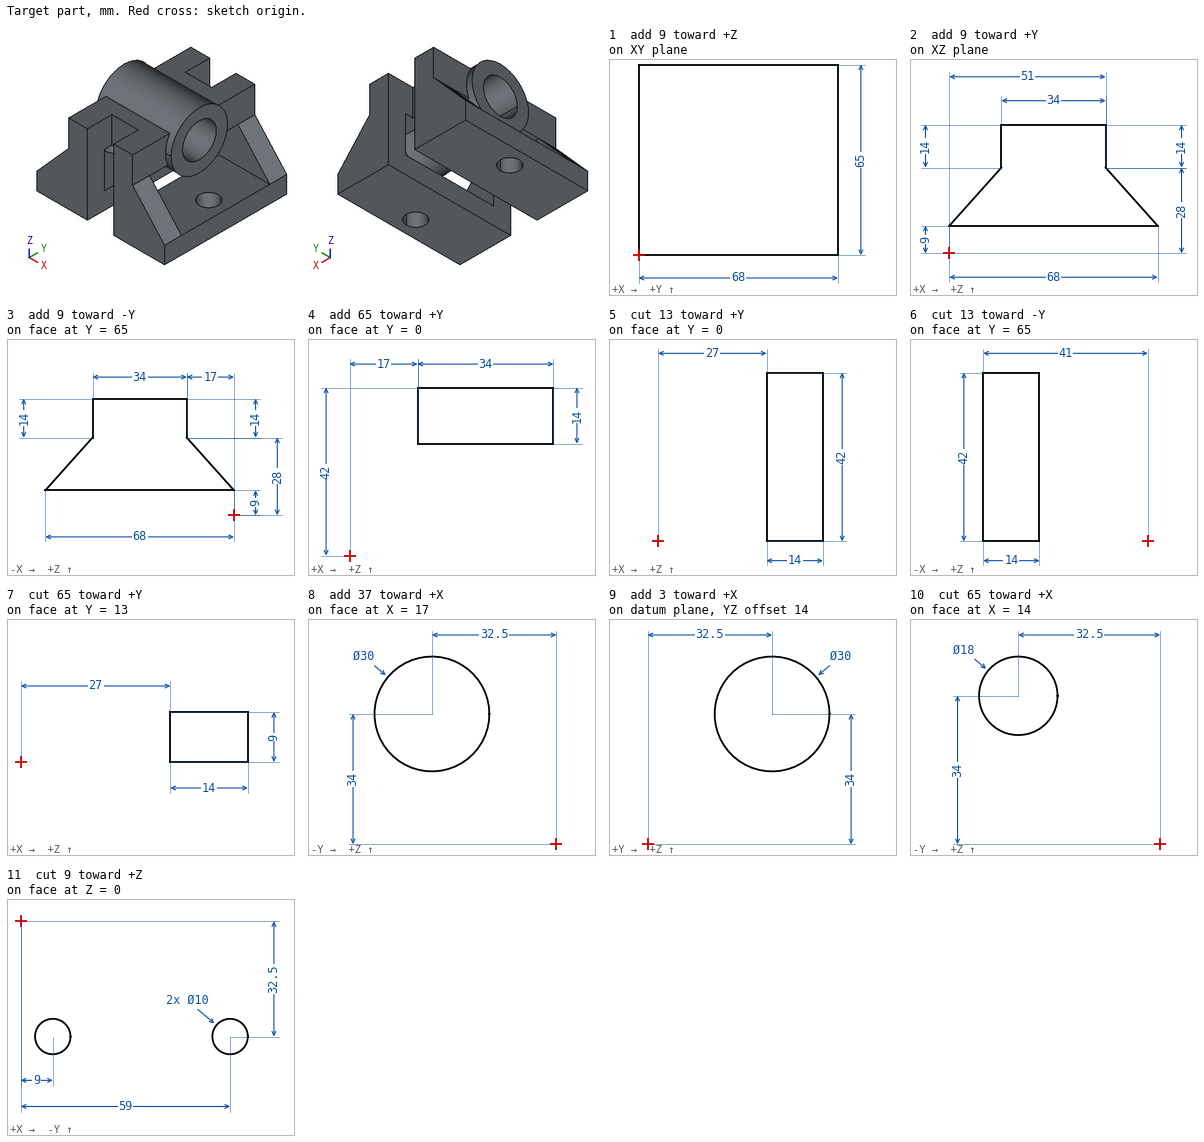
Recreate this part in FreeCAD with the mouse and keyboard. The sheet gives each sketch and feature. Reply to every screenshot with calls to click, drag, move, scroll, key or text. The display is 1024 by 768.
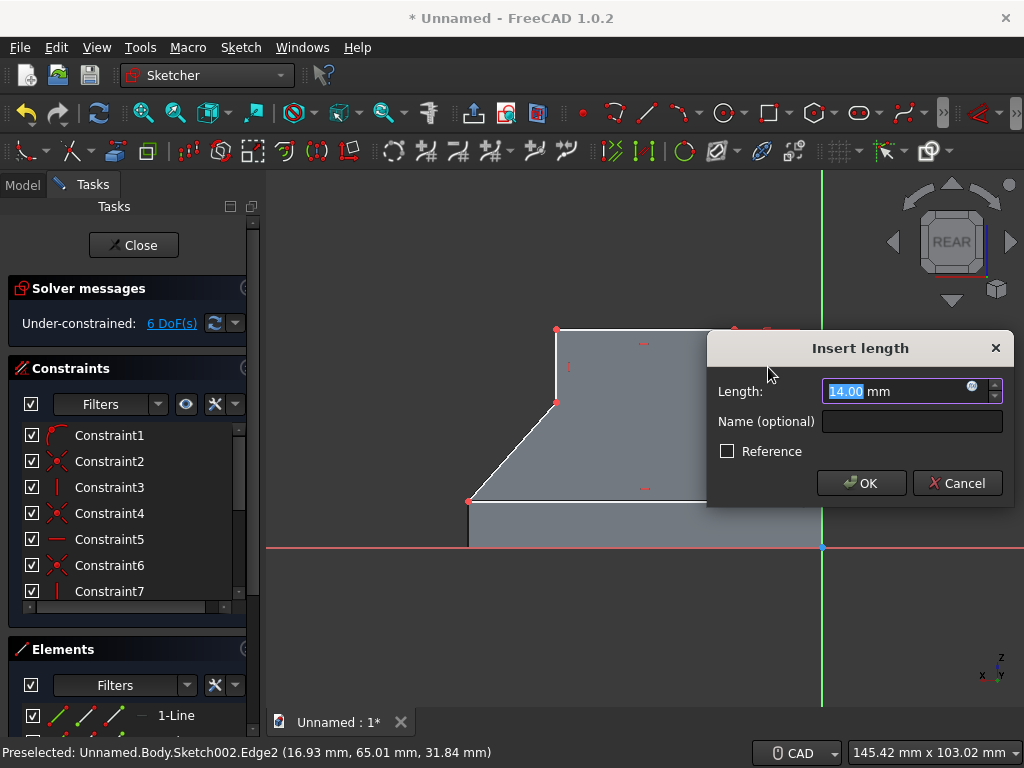
text(14)
key(Return)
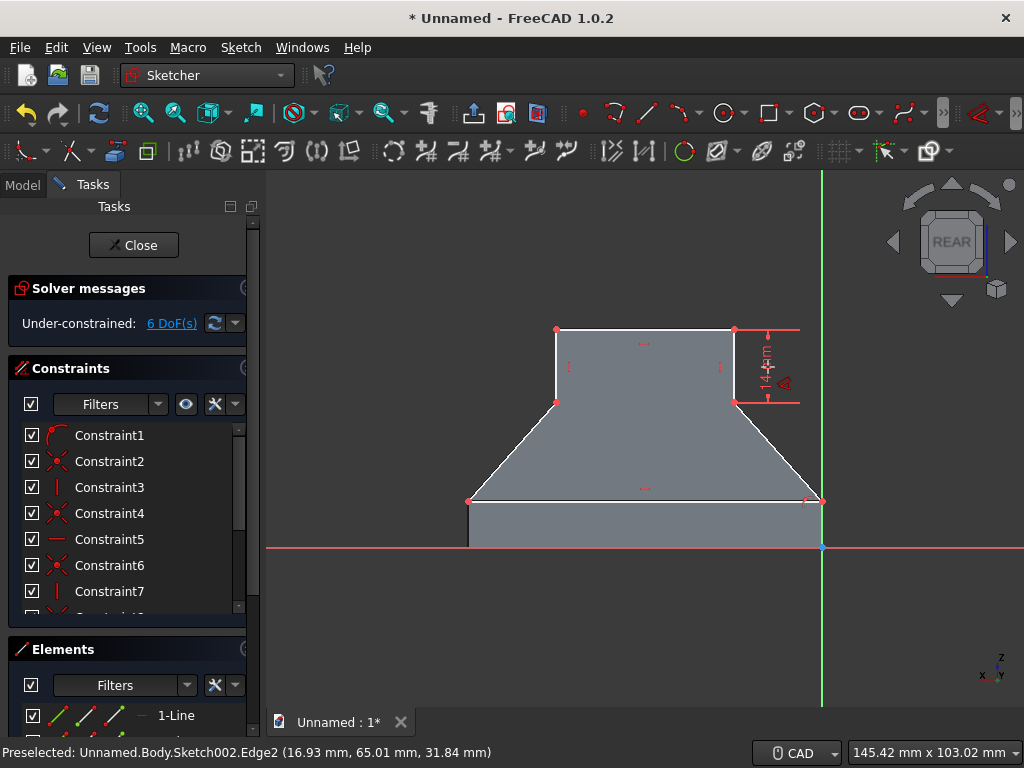
click(681, 330)
click(645, 296)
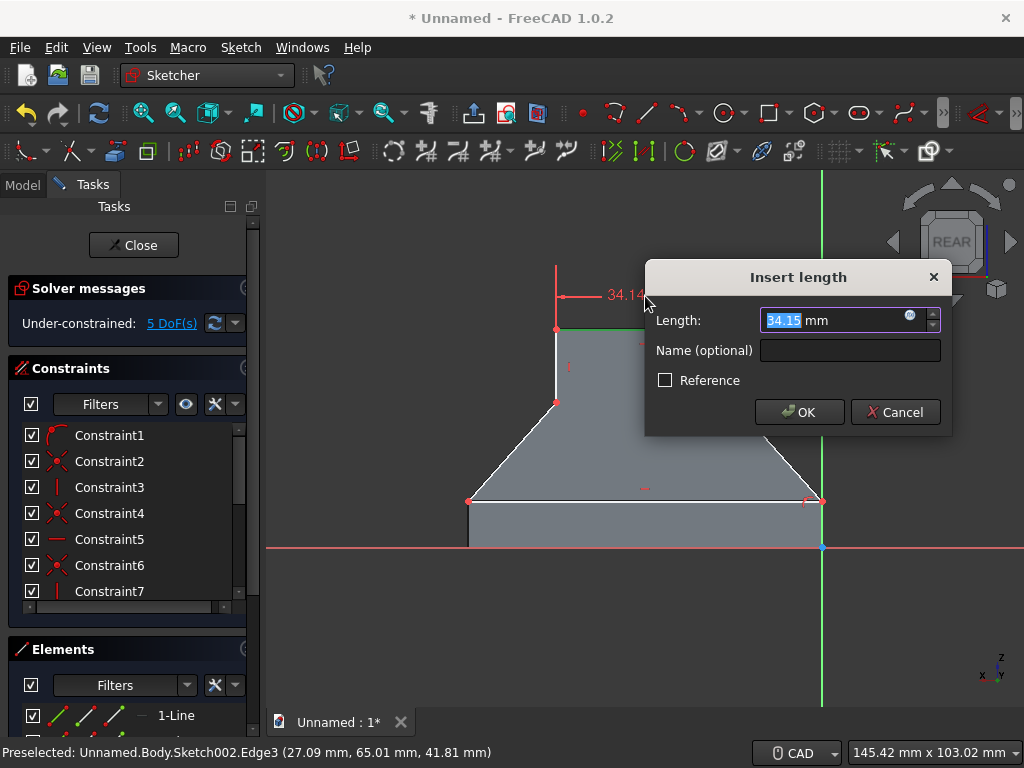
text(34)
key(Return)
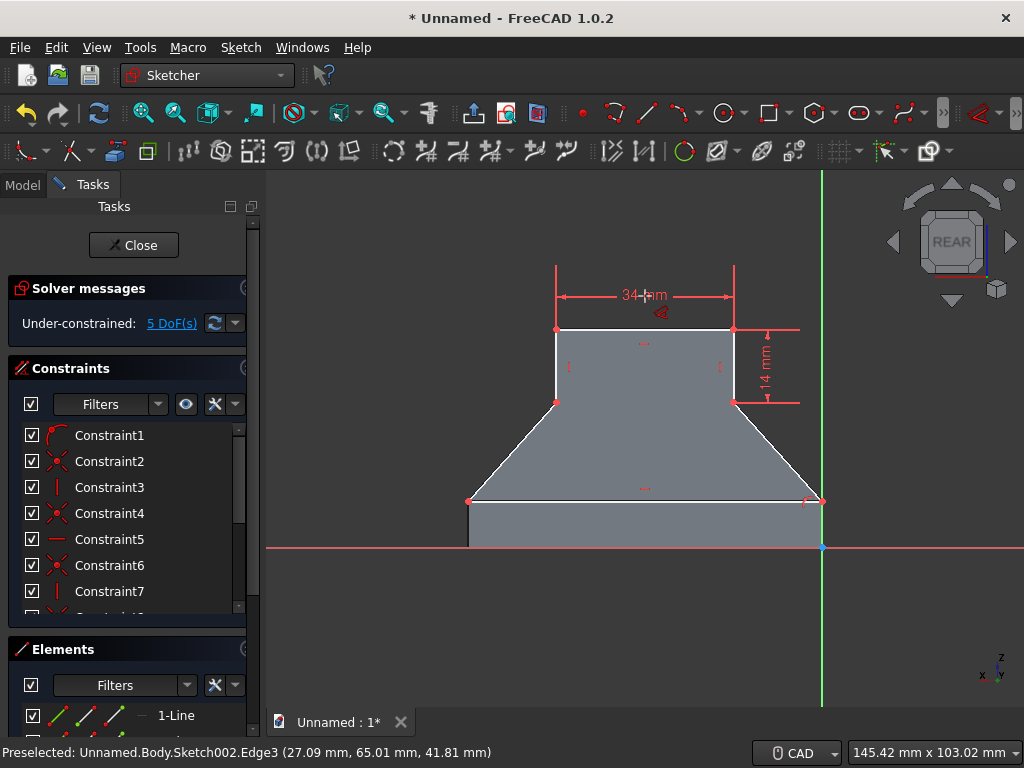
click(556, 352)
click(522, 367)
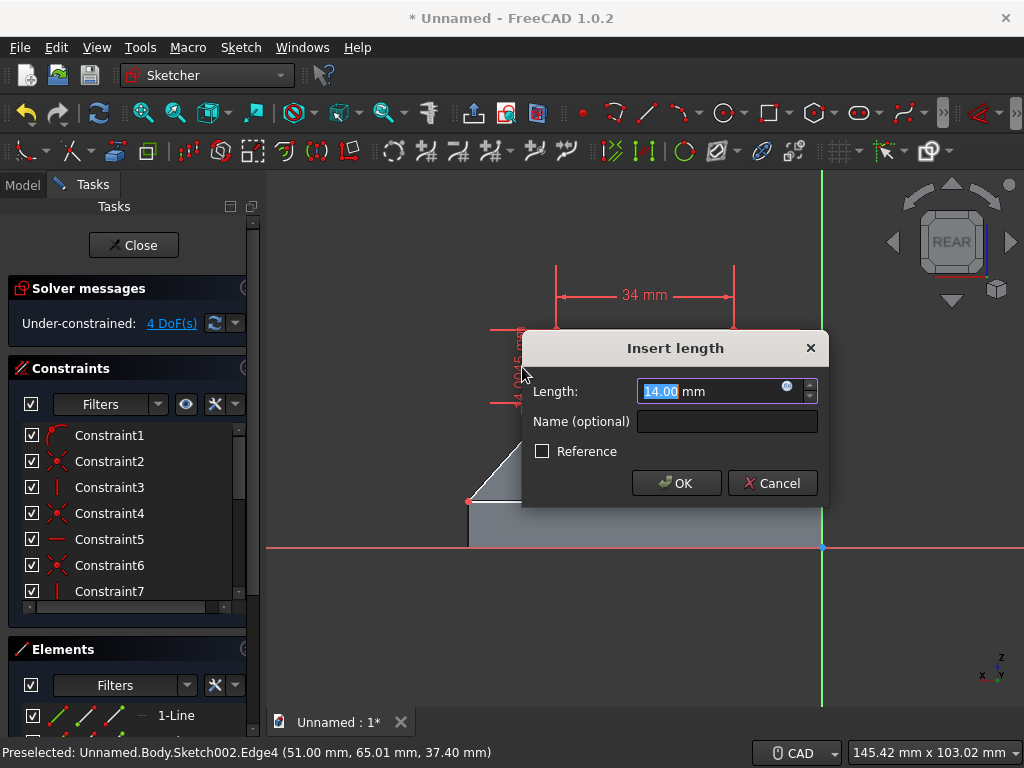
text(14)
key(Return)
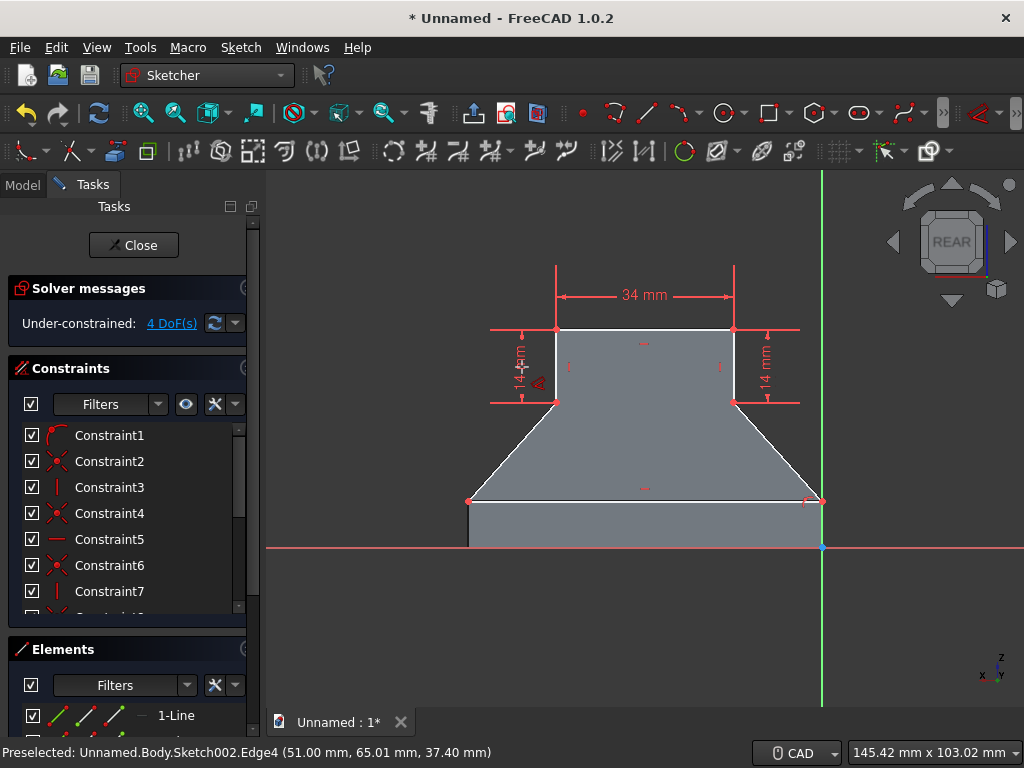
click(574, 502)
click(645, 468)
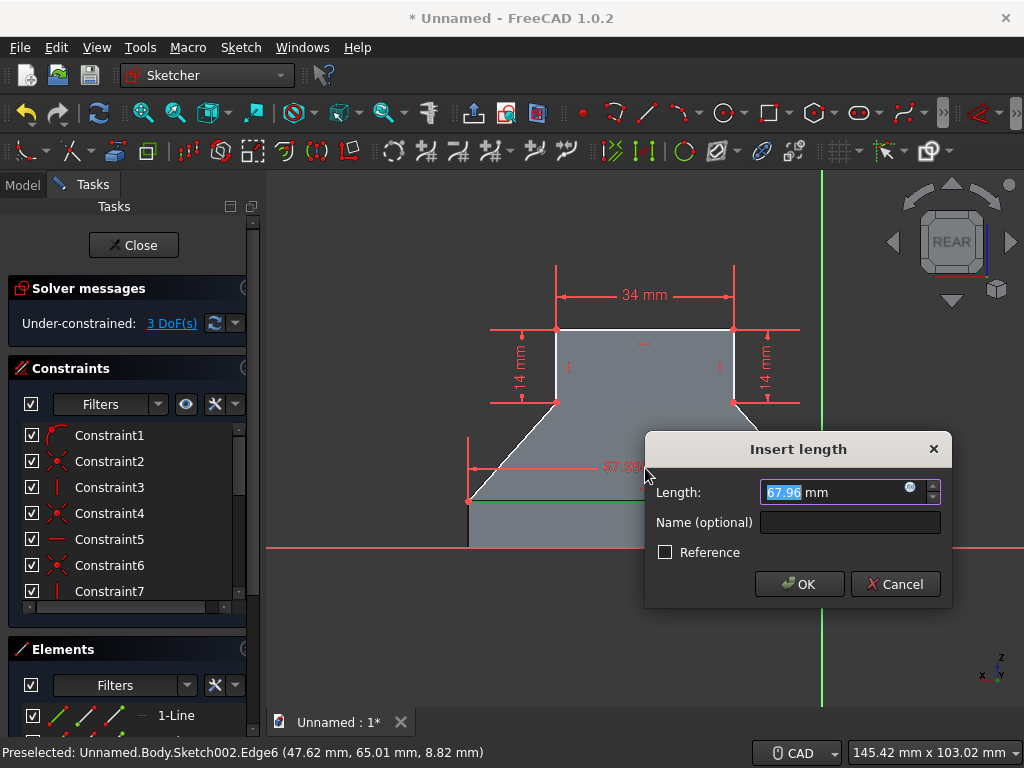
text(68)
key(Return)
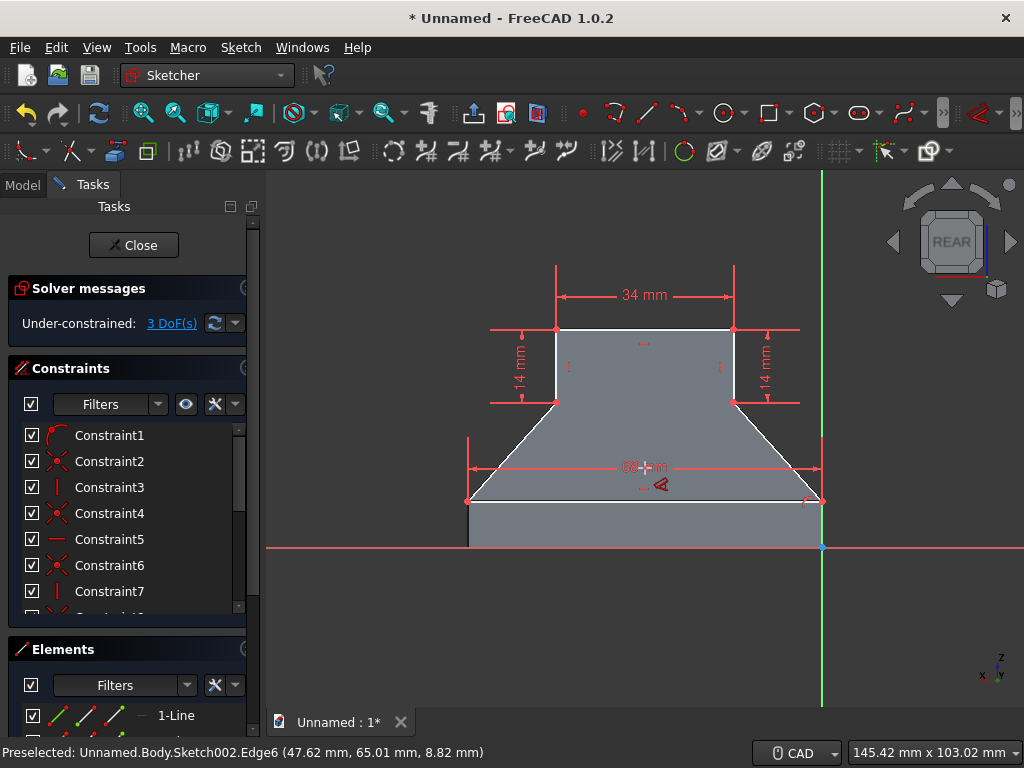
click(822, 502)
click(856, 525)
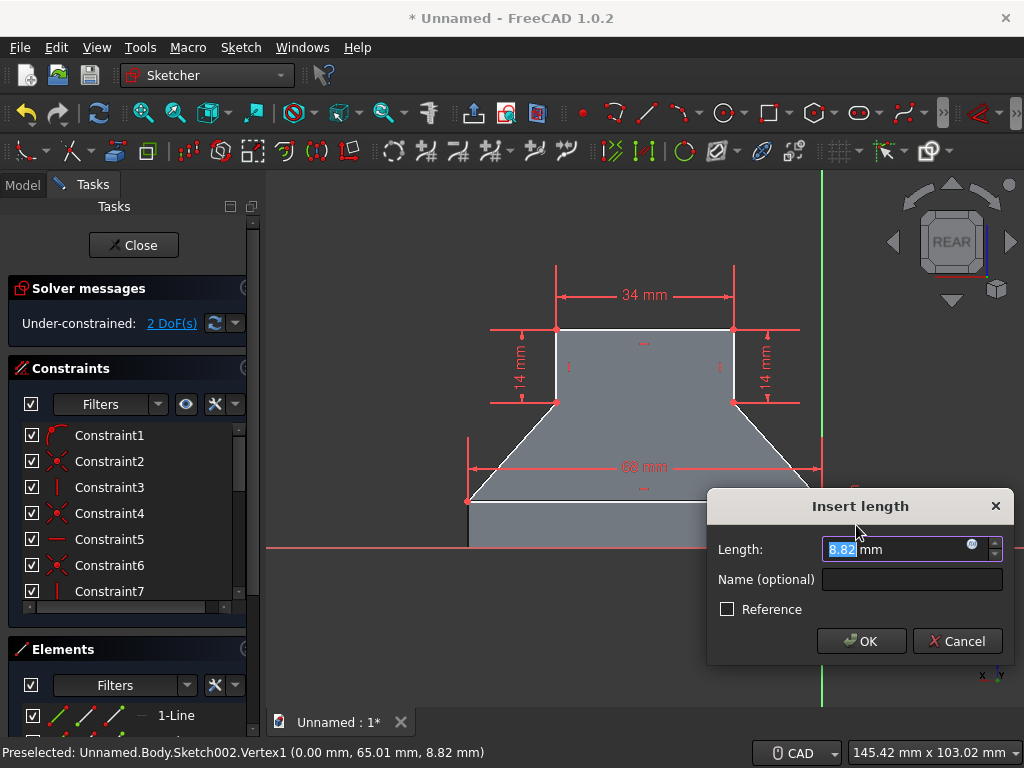
text(9)
key(Return)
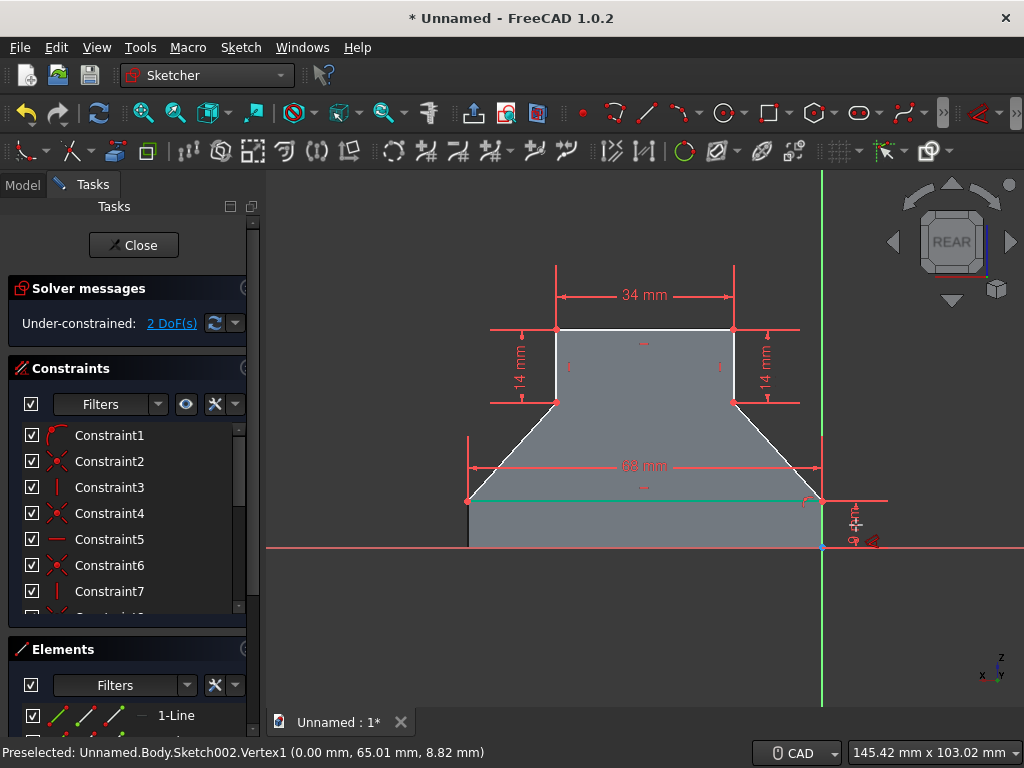
click(734, 403)
click(778, 582)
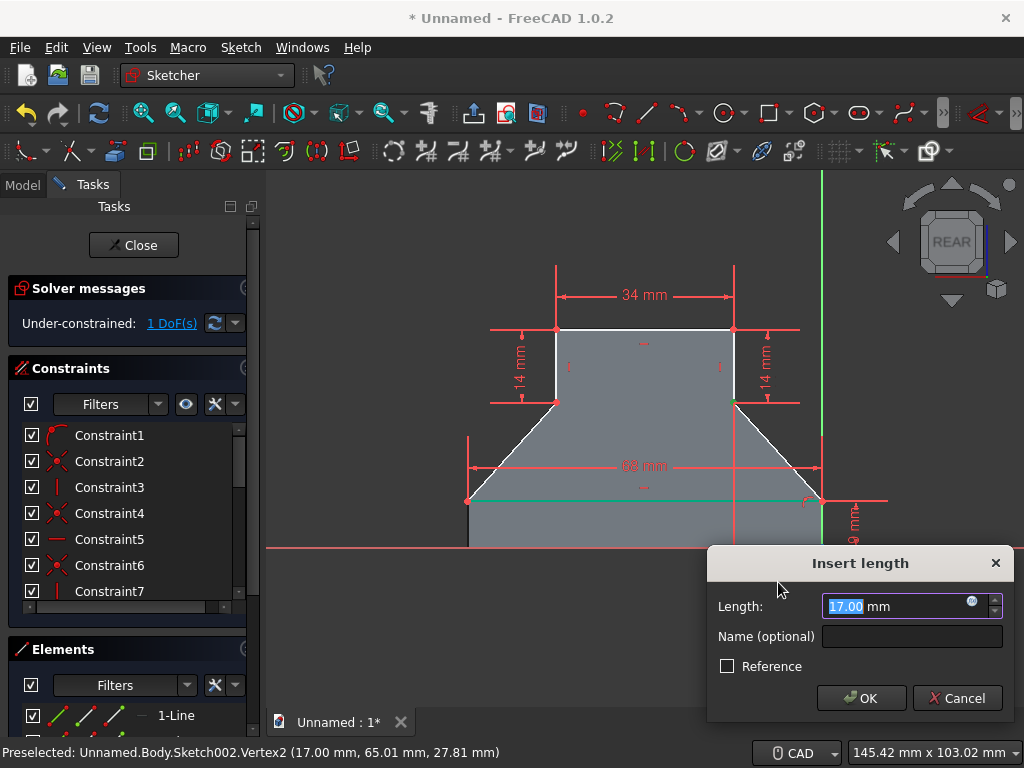
text(17)
key(Return)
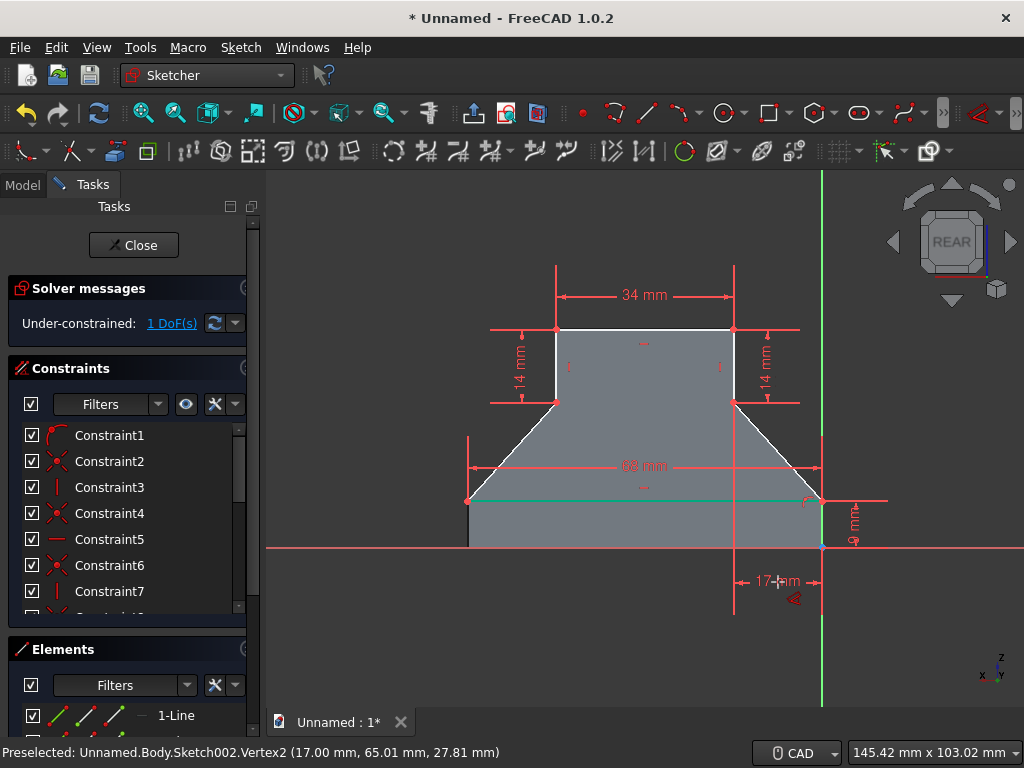
click(734, 403)
click(856, 475)